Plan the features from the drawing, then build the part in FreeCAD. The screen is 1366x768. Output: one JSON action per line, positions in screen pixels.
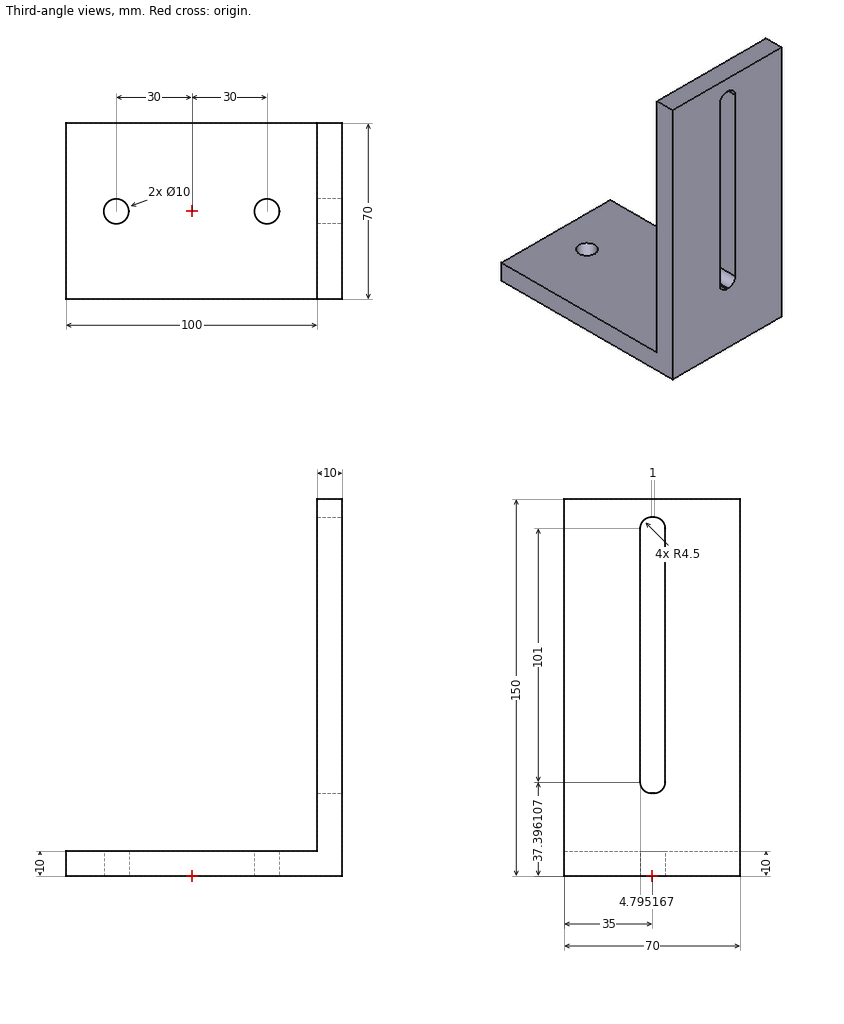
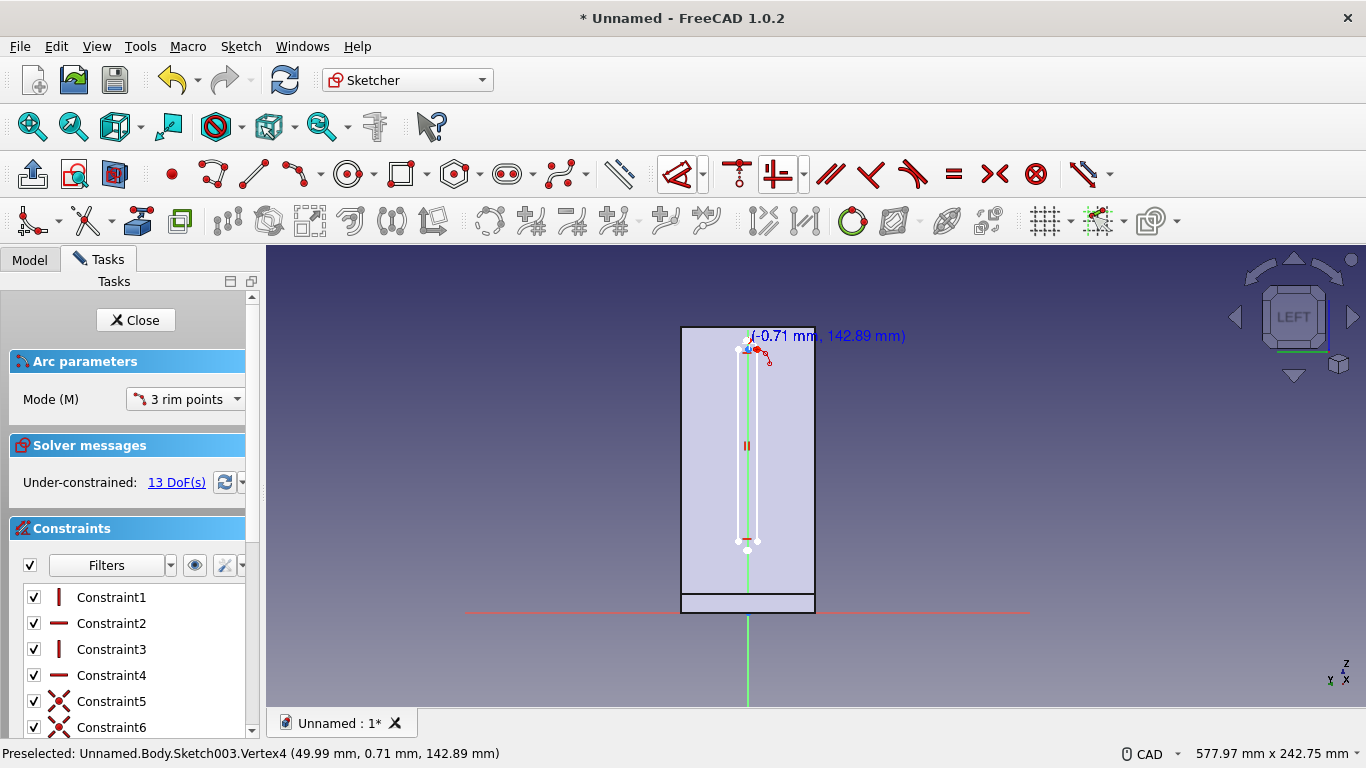
{"action": "scroll", "coordinate": [738, 349], "scroll_direction": "up", "scroll_amount": 3}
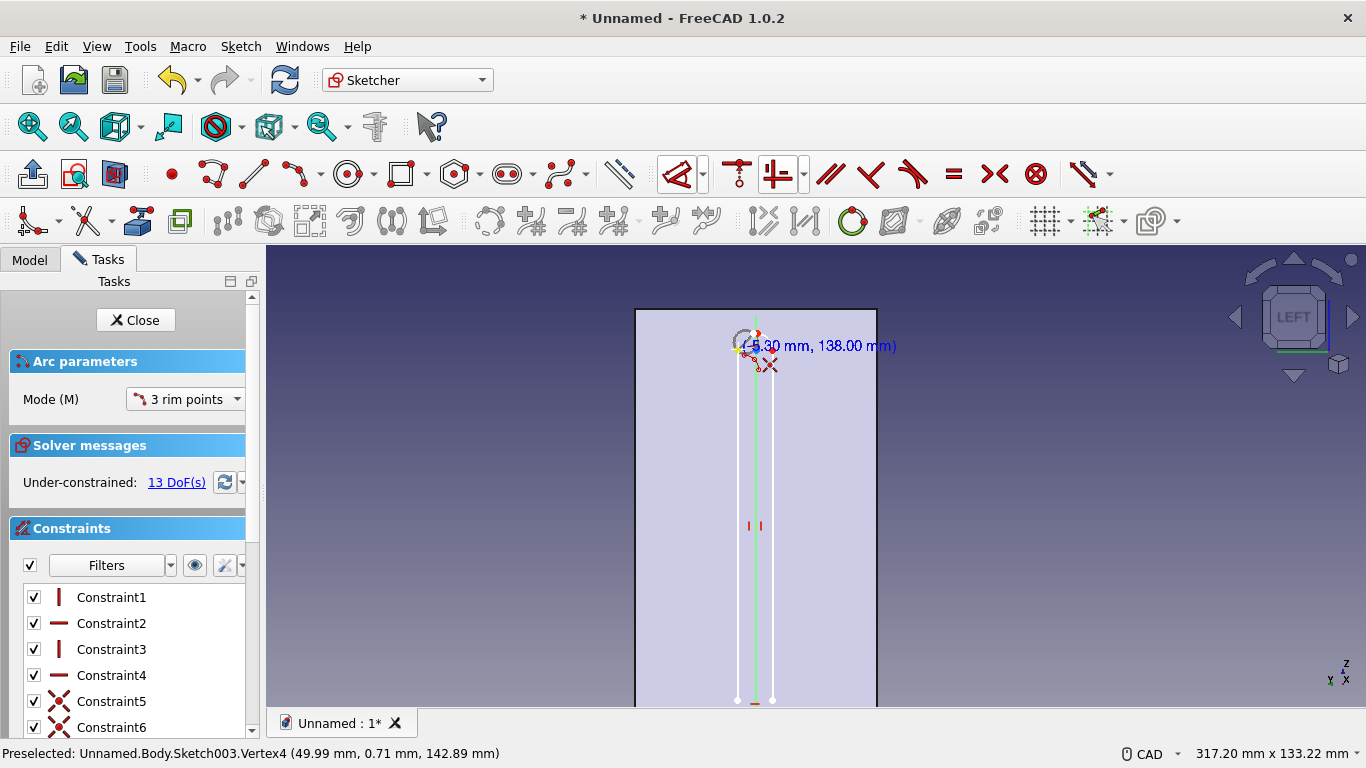
{"action": "left_click", "coordinate": [738, 350]}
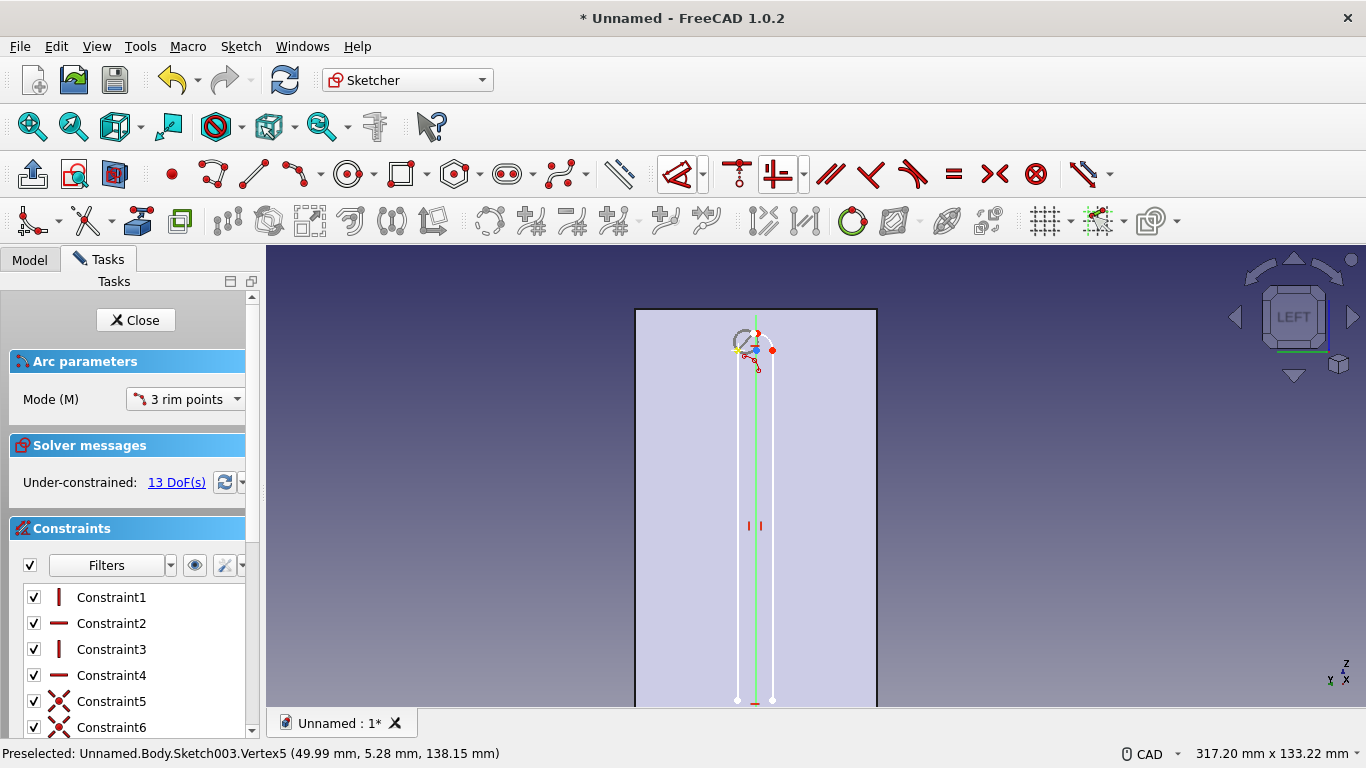
{"action": "scroll", "coordinate": [743, 338], "scroll_direction": "up", "scroll_amount": 7}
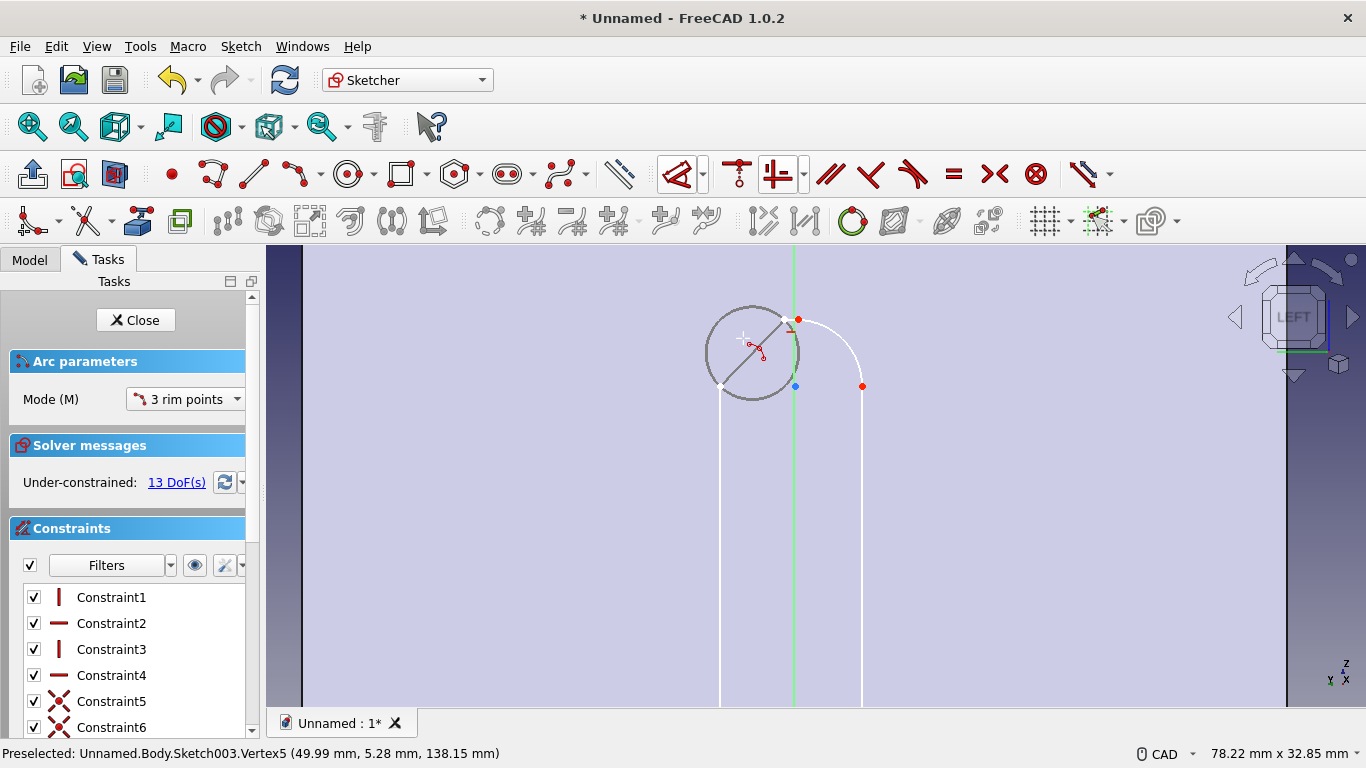
{"action": "left_click", "coordinate": [740, 338]}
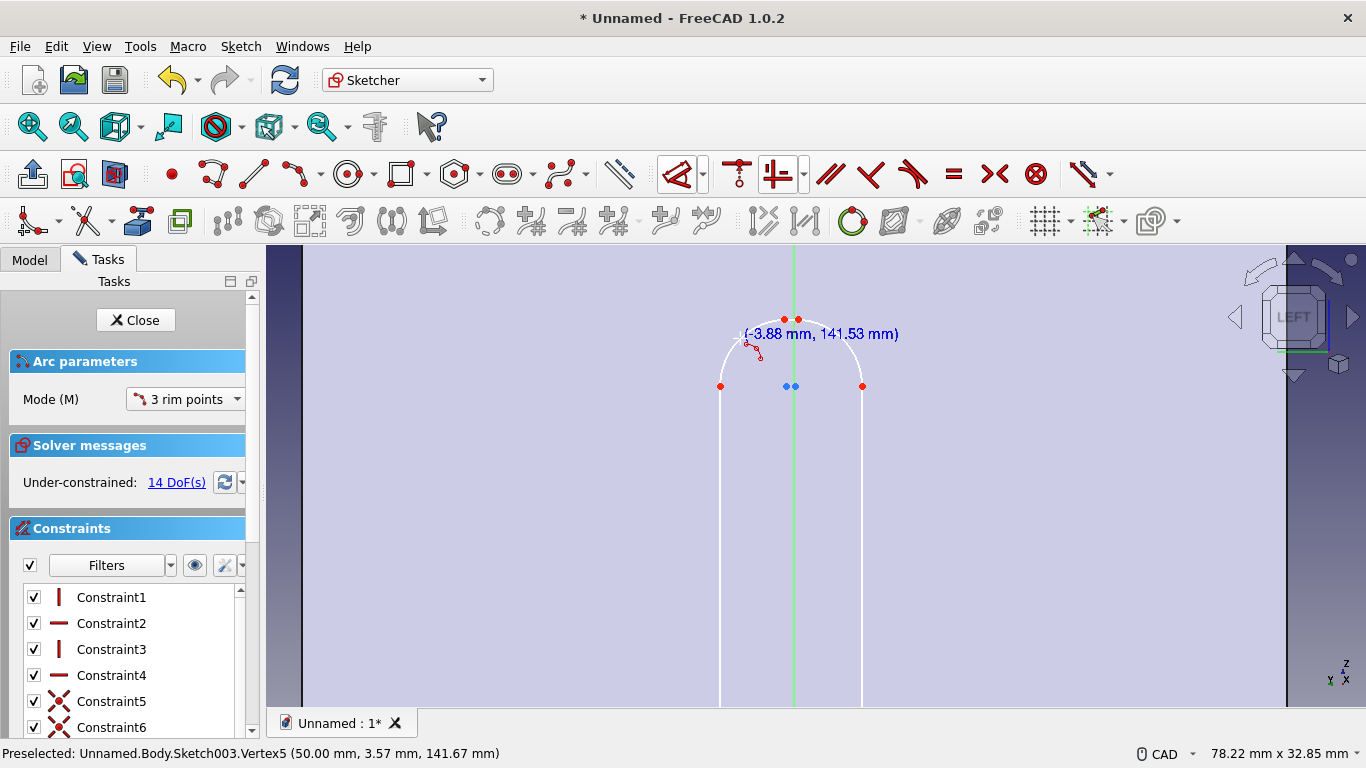
{"action": "scroll", "coordinate": [741, 343], "scroll_direction": "down", "scroll_amount": 10}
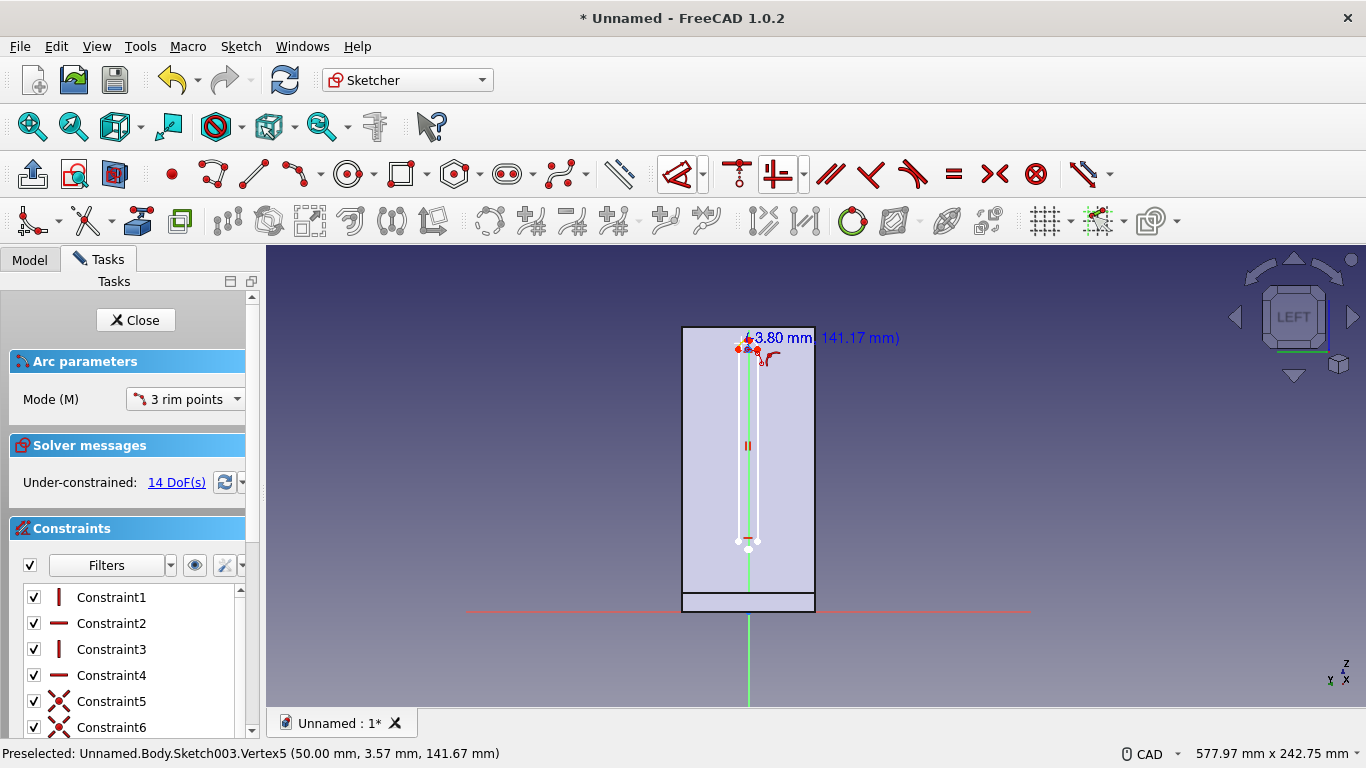
{"action": "scroll", "coordinate": [739, 541], "scroll_direction": "up", "scroll_amount": 3}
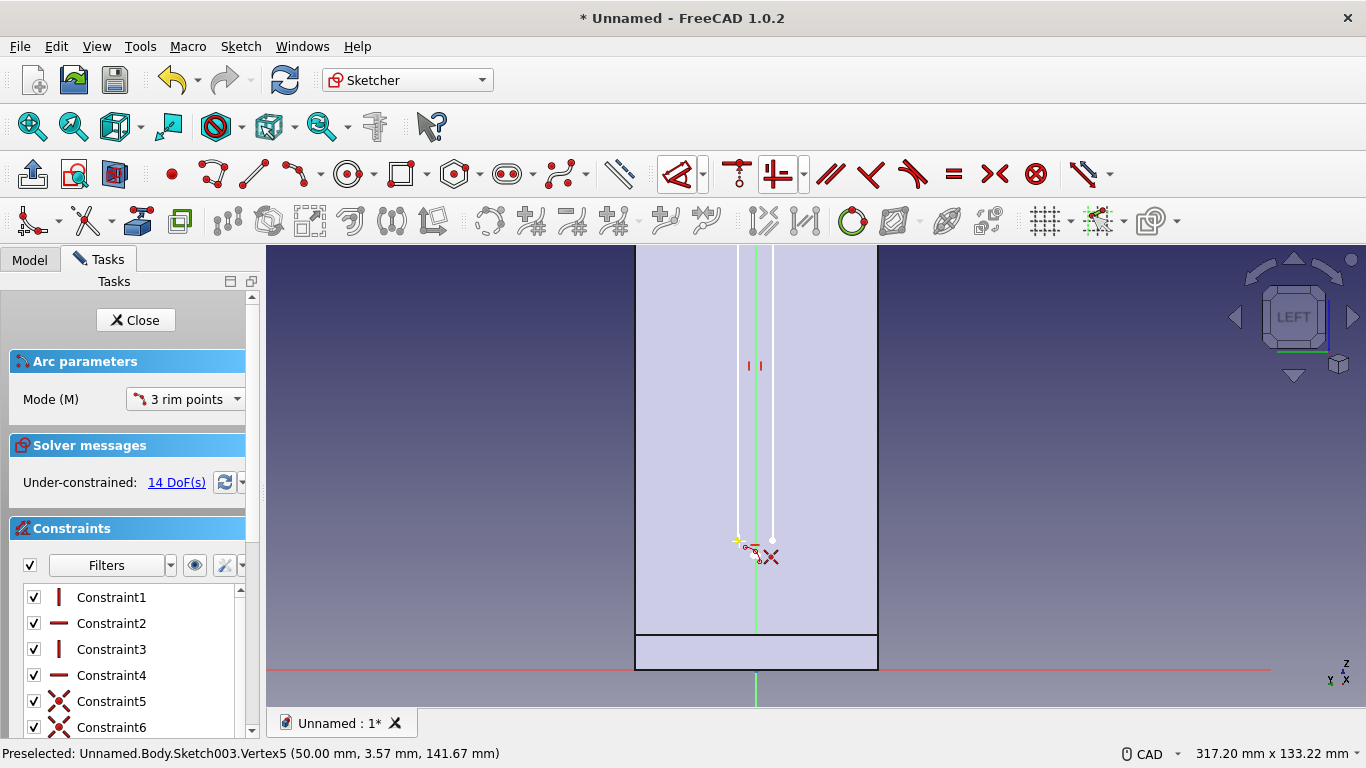
{"action": "left_click", "coordinate": [738, 541]}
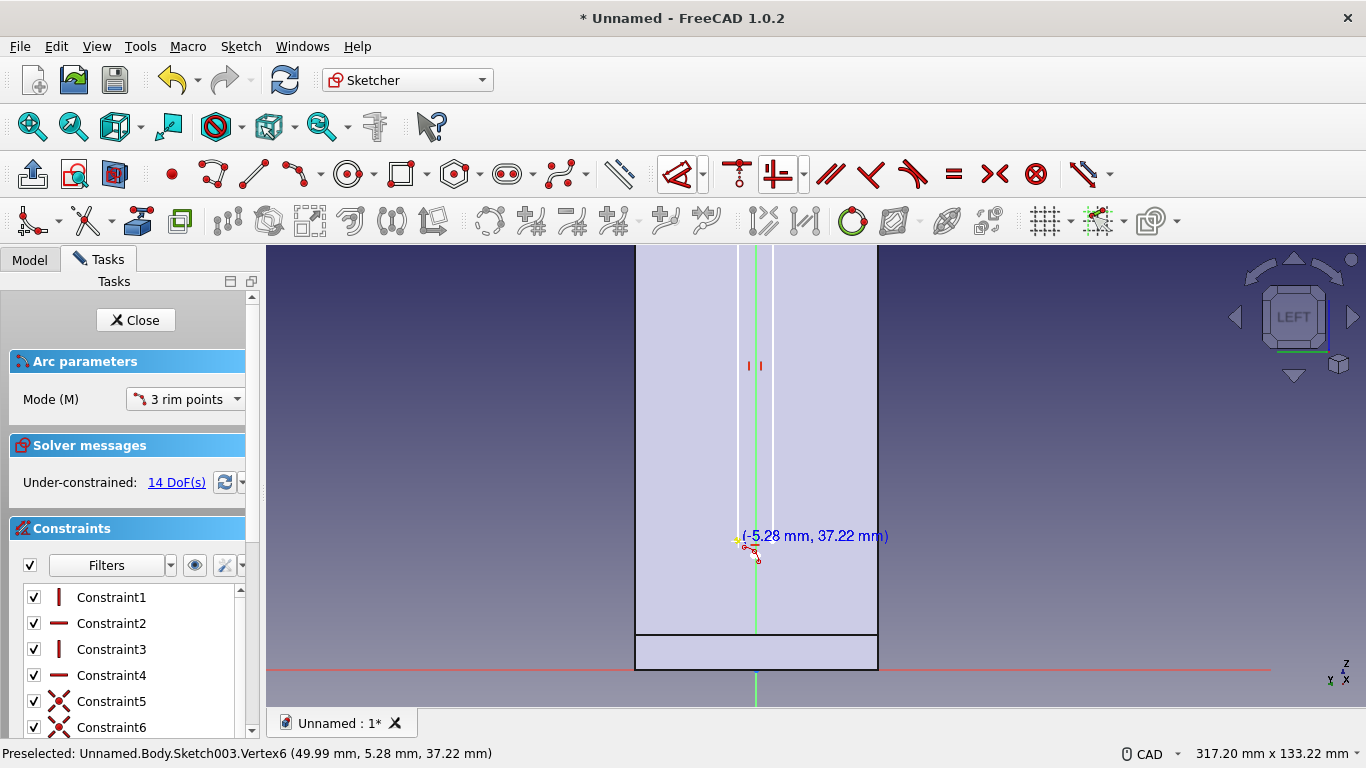
{"action": "scroll", "coordinate": [754, 556], "scroll_direction": "up", "scroll_amount": 12}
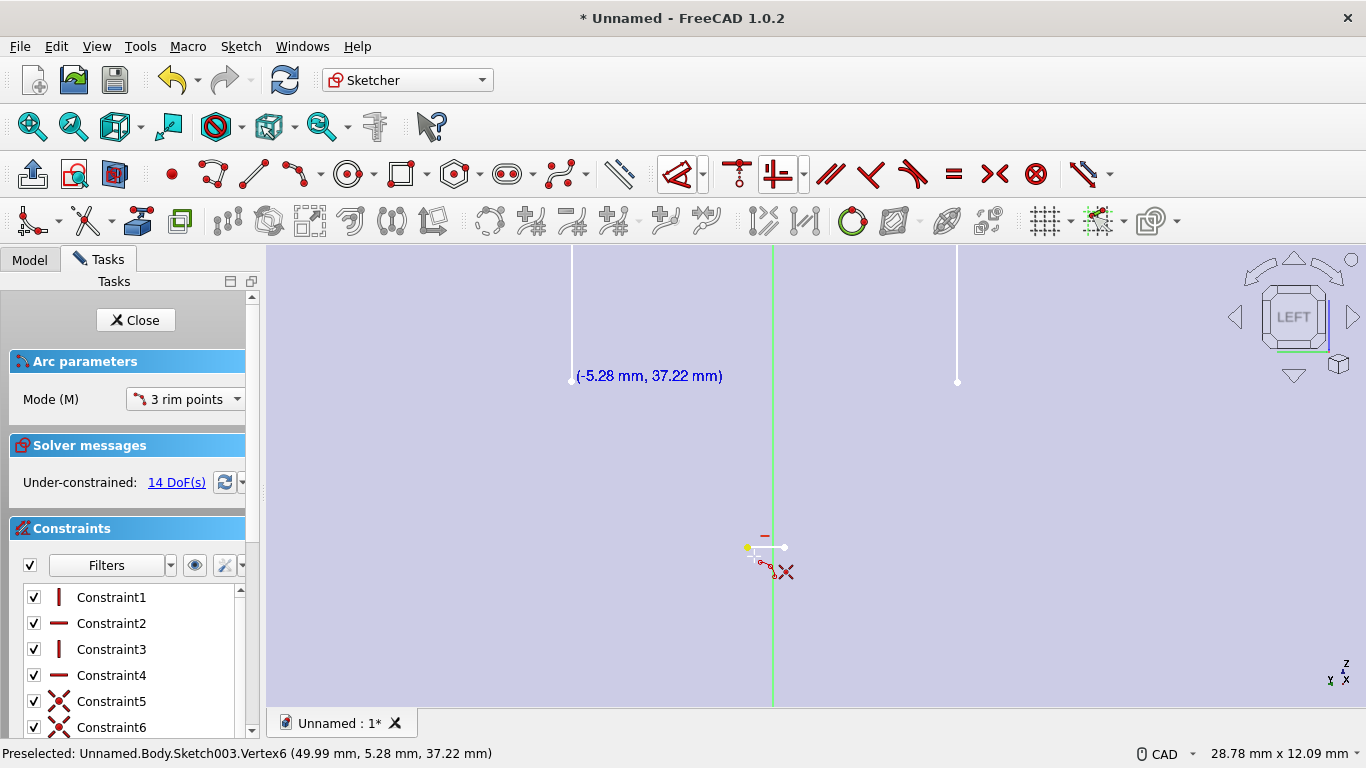
{"action": "left_click", "coordinate": [747, 547]}